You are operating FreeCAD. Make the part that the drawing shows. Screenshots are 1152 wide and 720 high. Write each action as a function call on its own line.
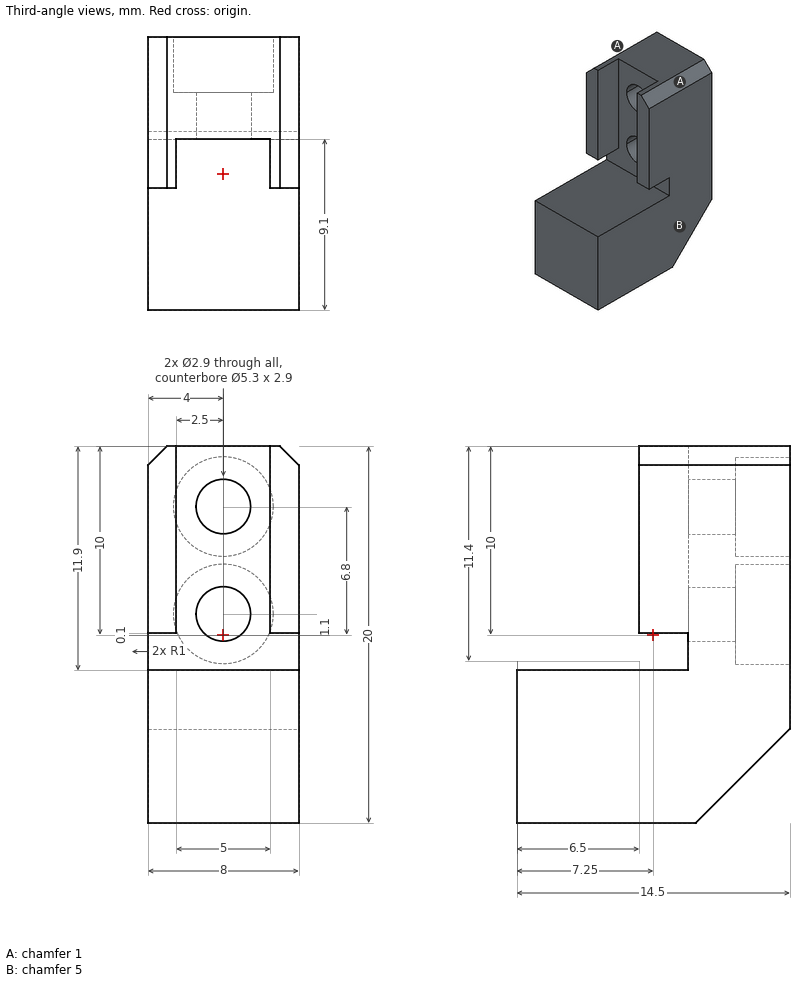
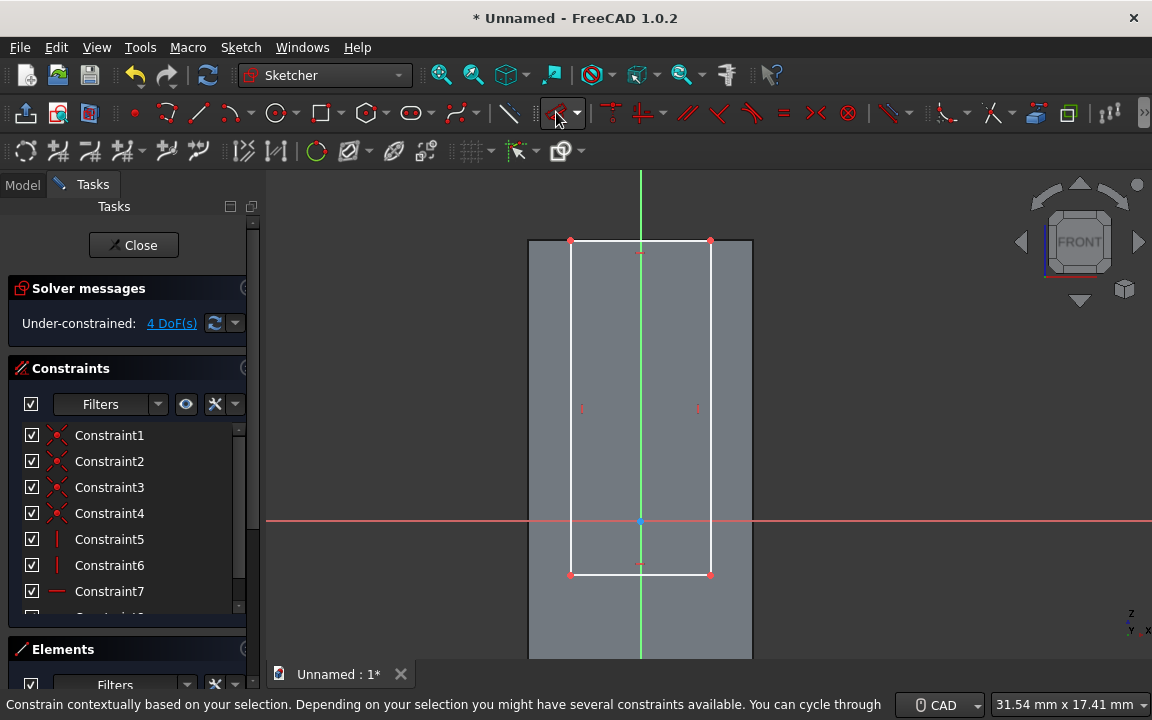
click(613, 575)
click(608, 609)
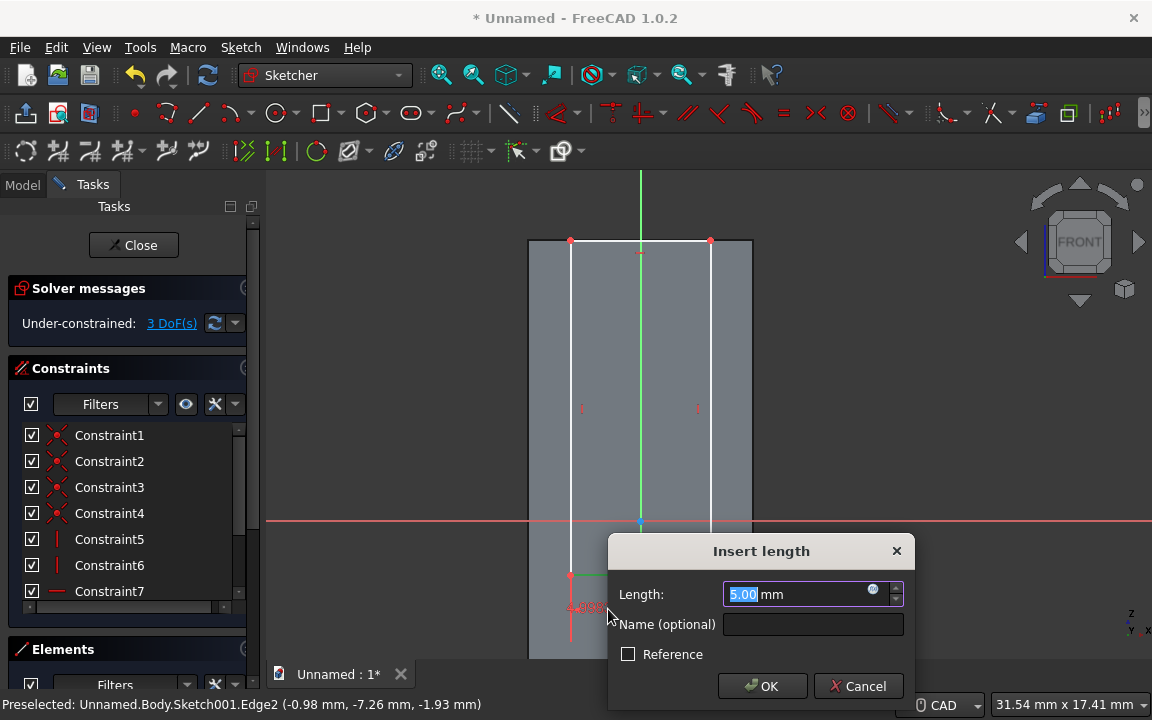
text(5)
key(Return)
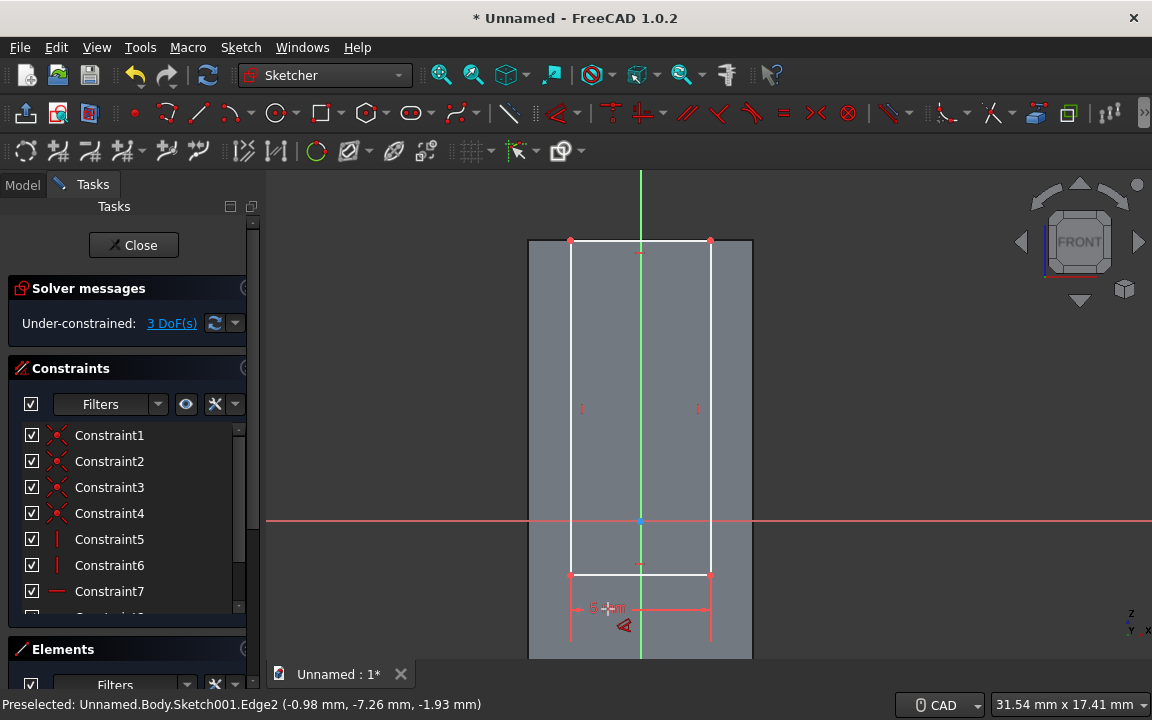
click(571, 241)
click(537, 381)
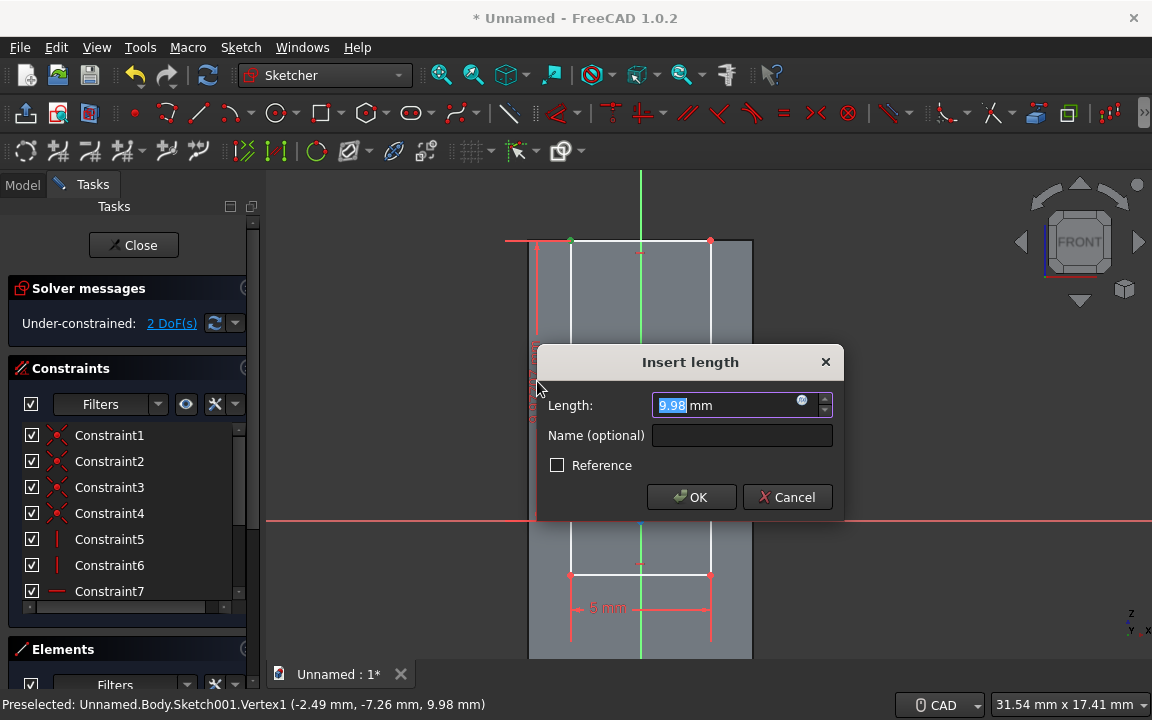
text(10)
key(Return)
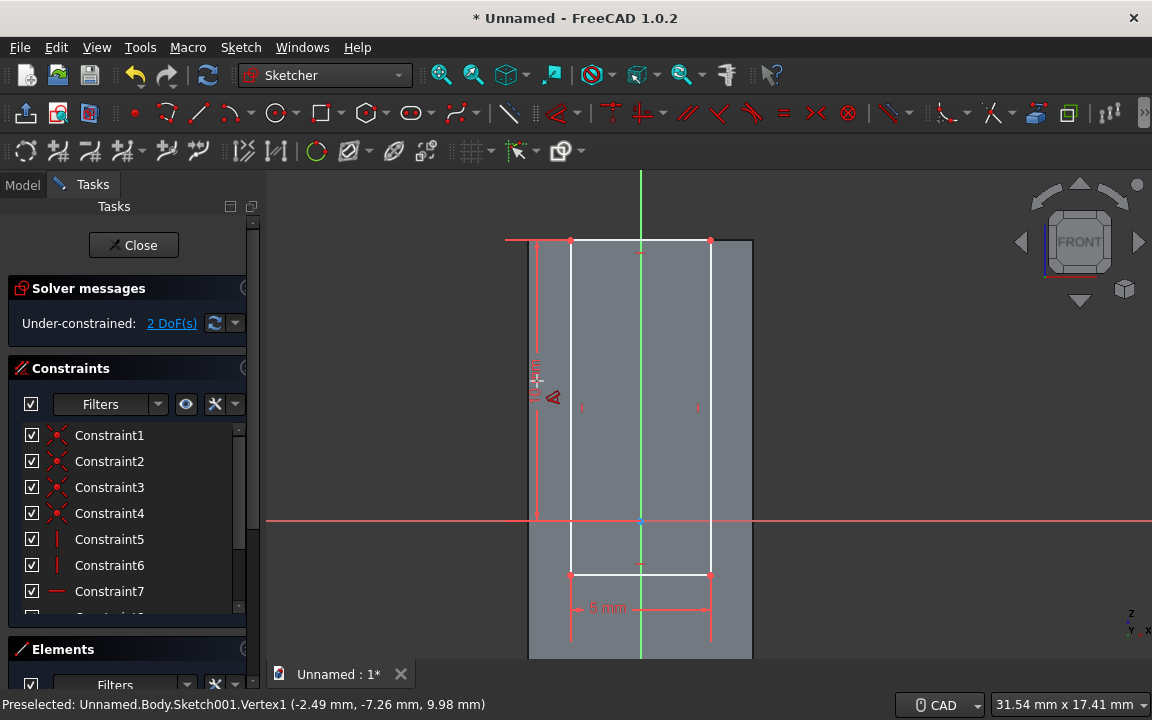
click(571, 341)
click(537, 408)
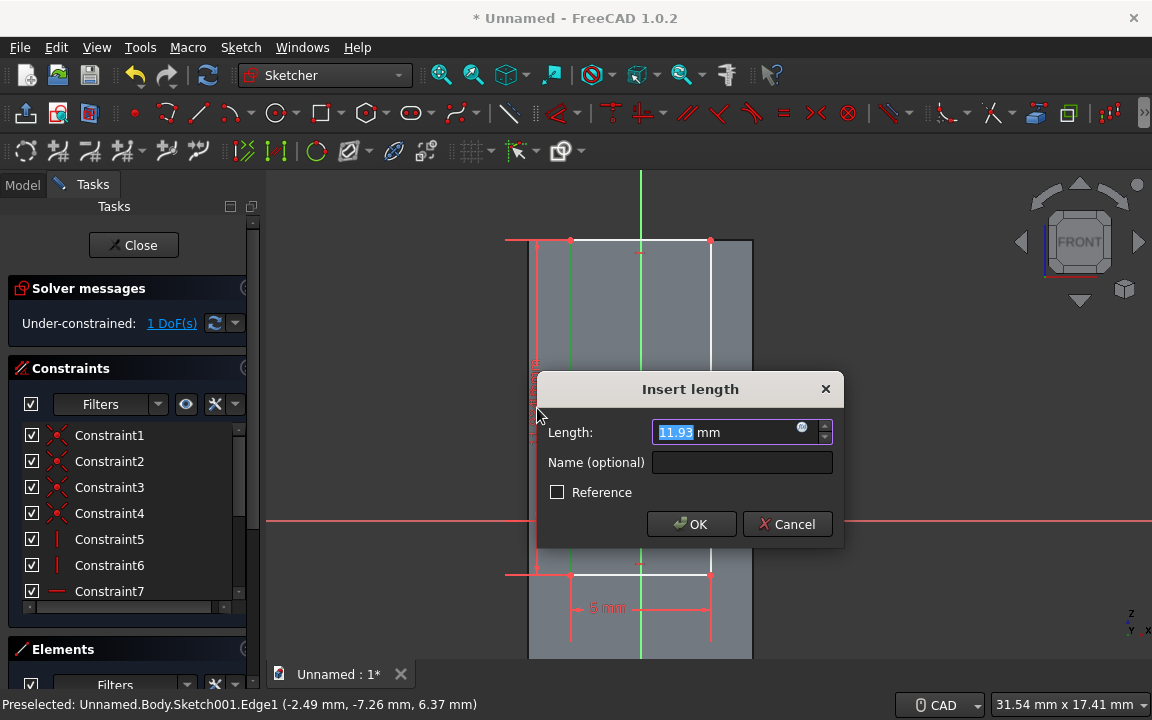
text(11.9)
key(Return)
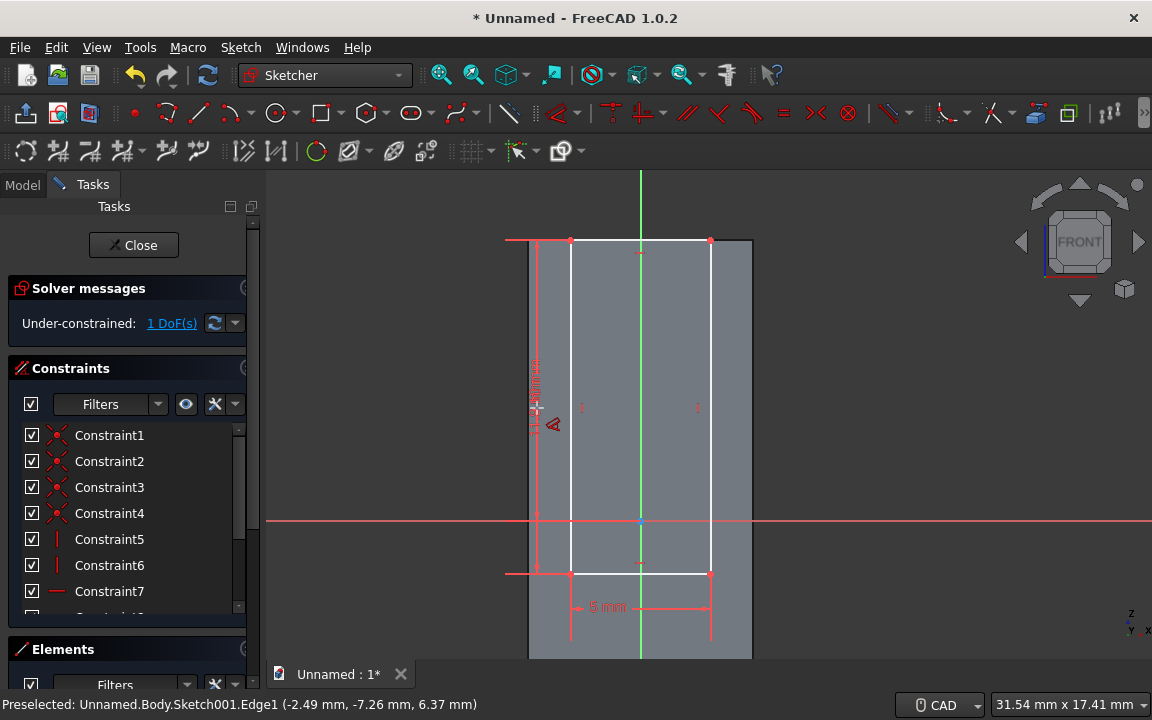
click(571, 240)
click(606, 206)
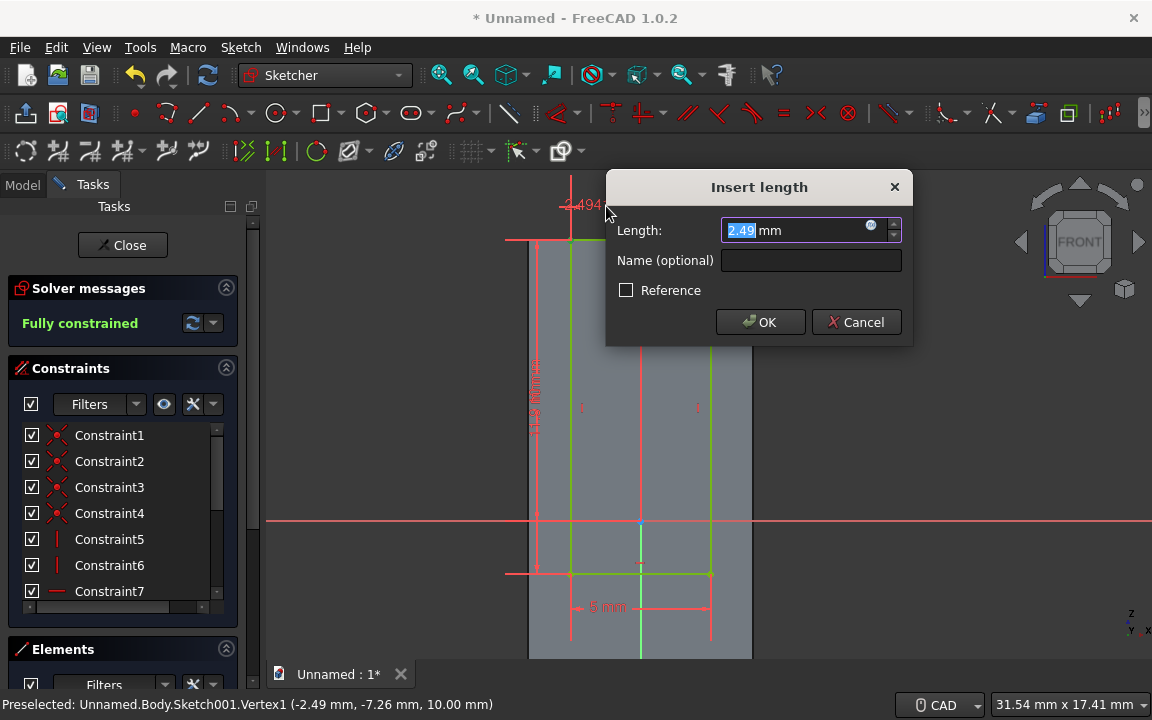
text(2.5)
key(Return)
key(Escape)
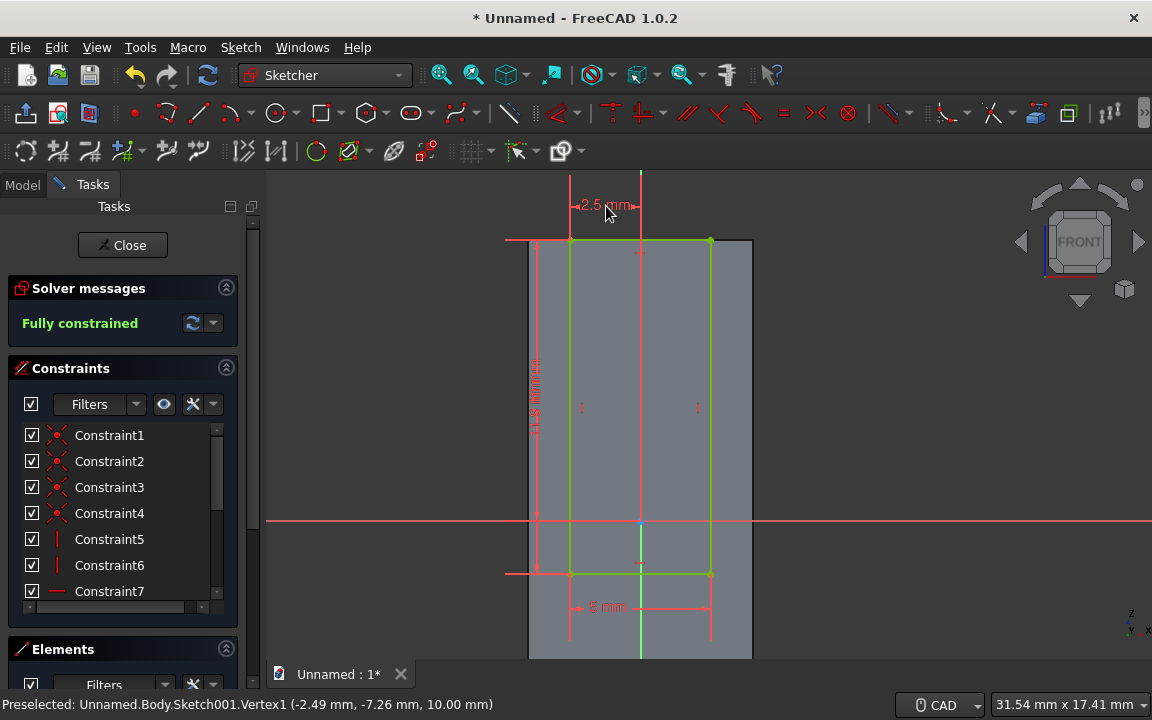
click(123, 245)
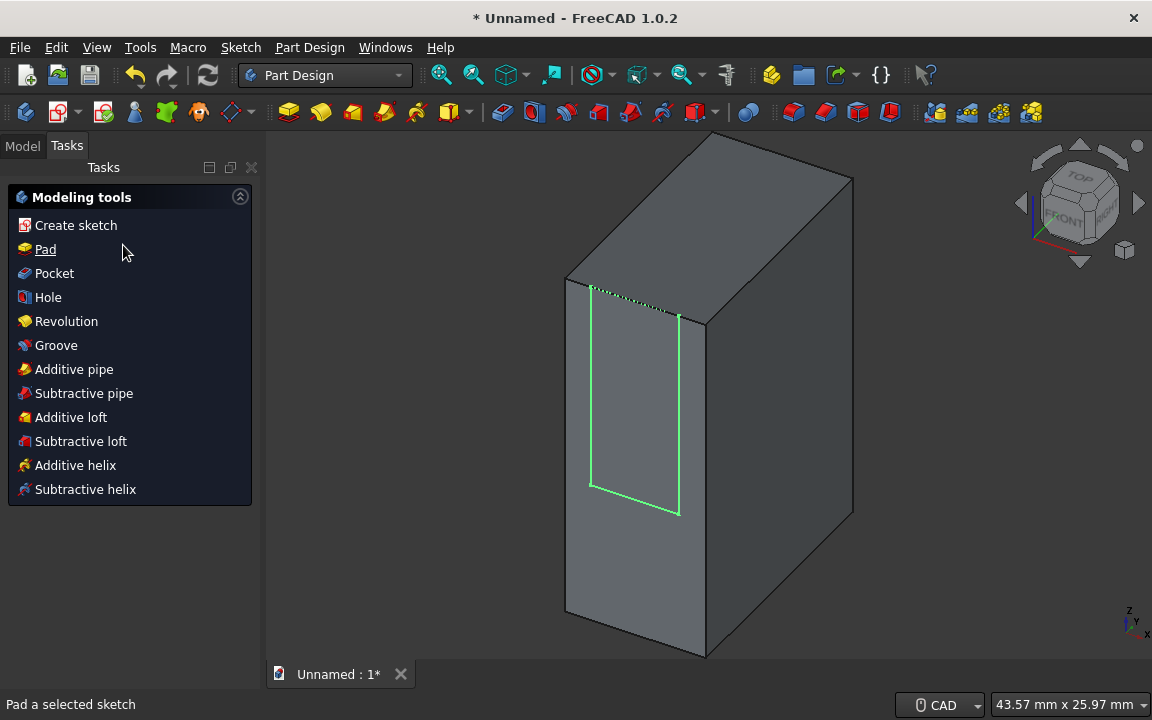
click(504, 112)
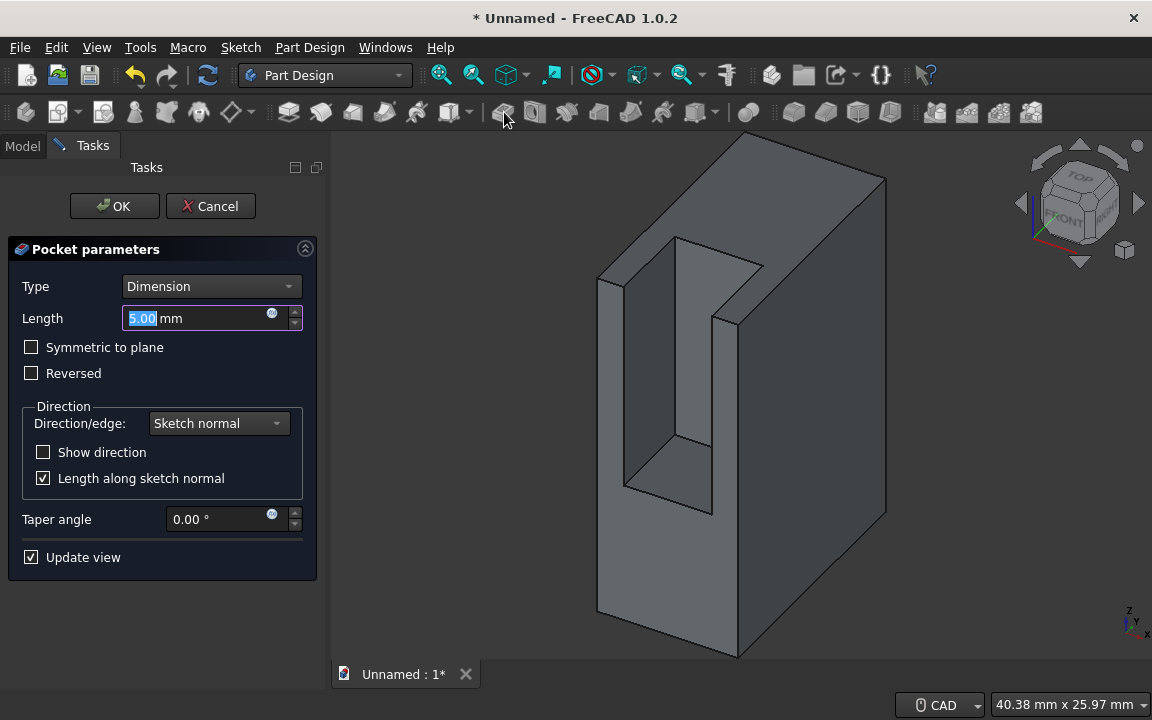
text(9.1)
key(Tab)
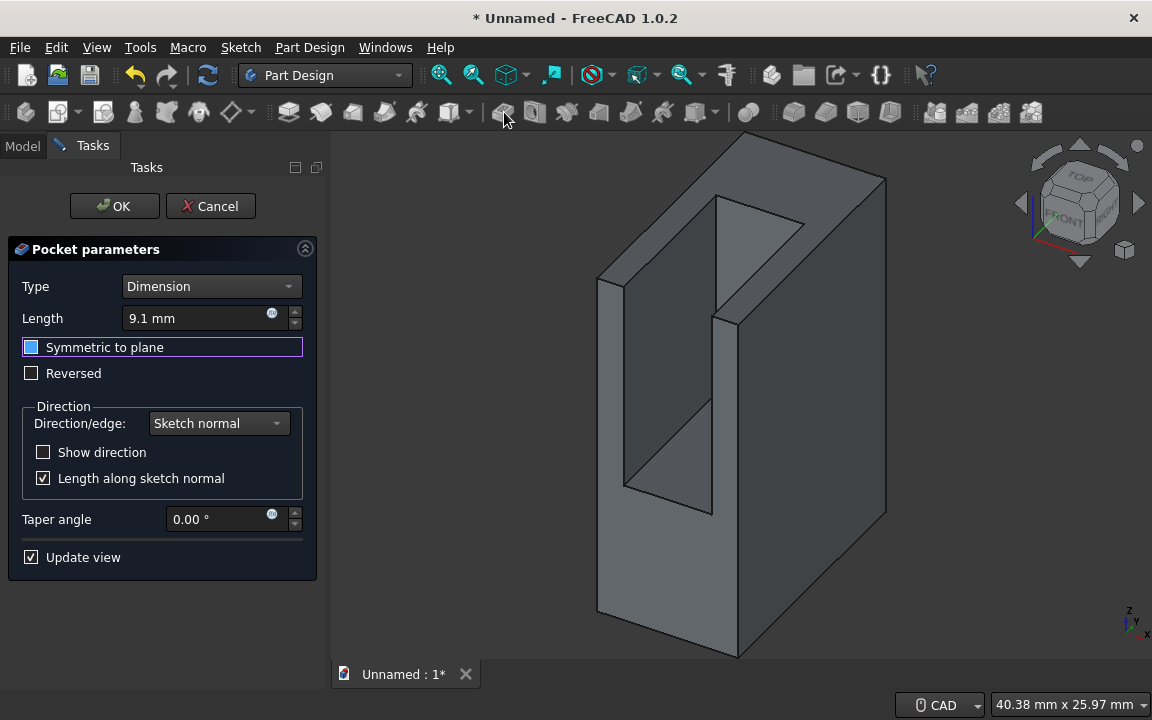
click(115, 206)